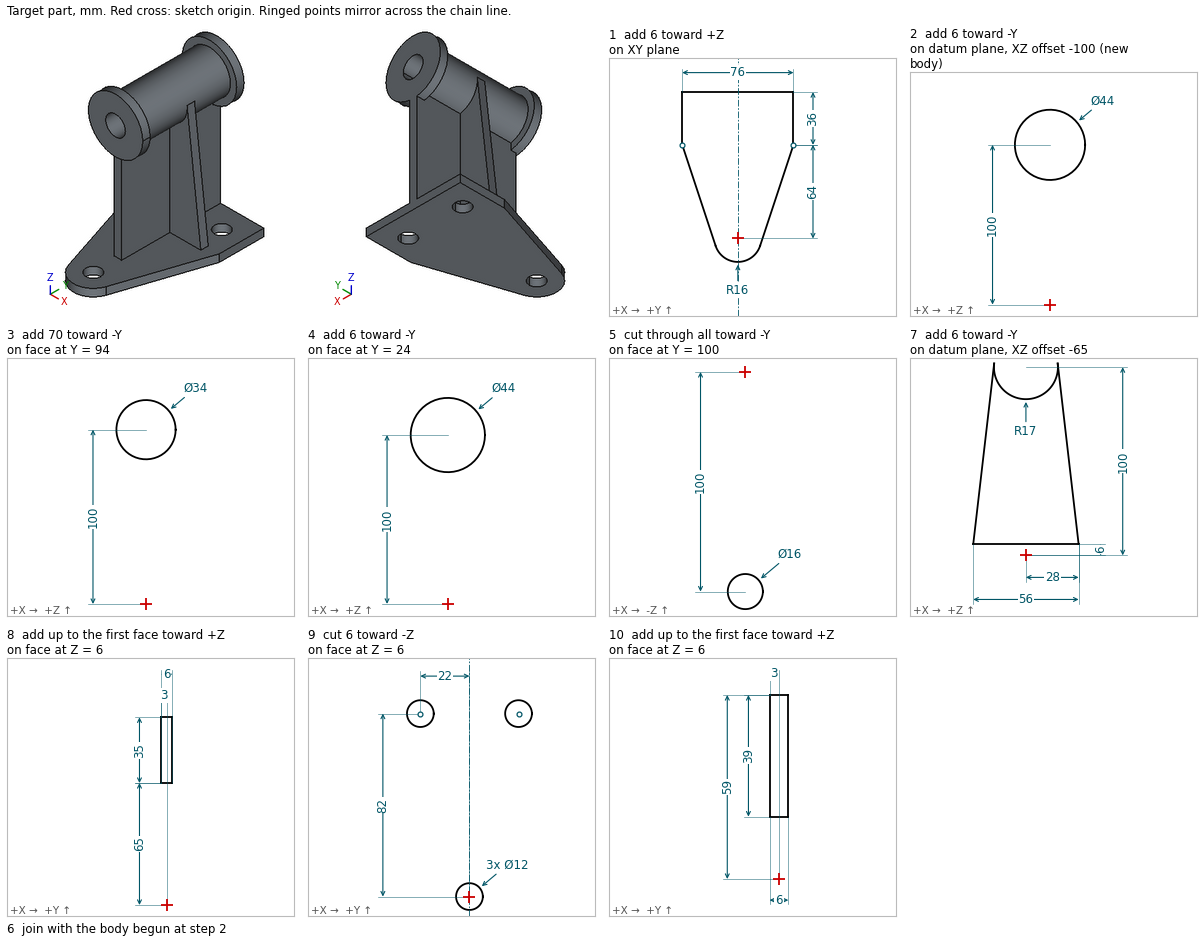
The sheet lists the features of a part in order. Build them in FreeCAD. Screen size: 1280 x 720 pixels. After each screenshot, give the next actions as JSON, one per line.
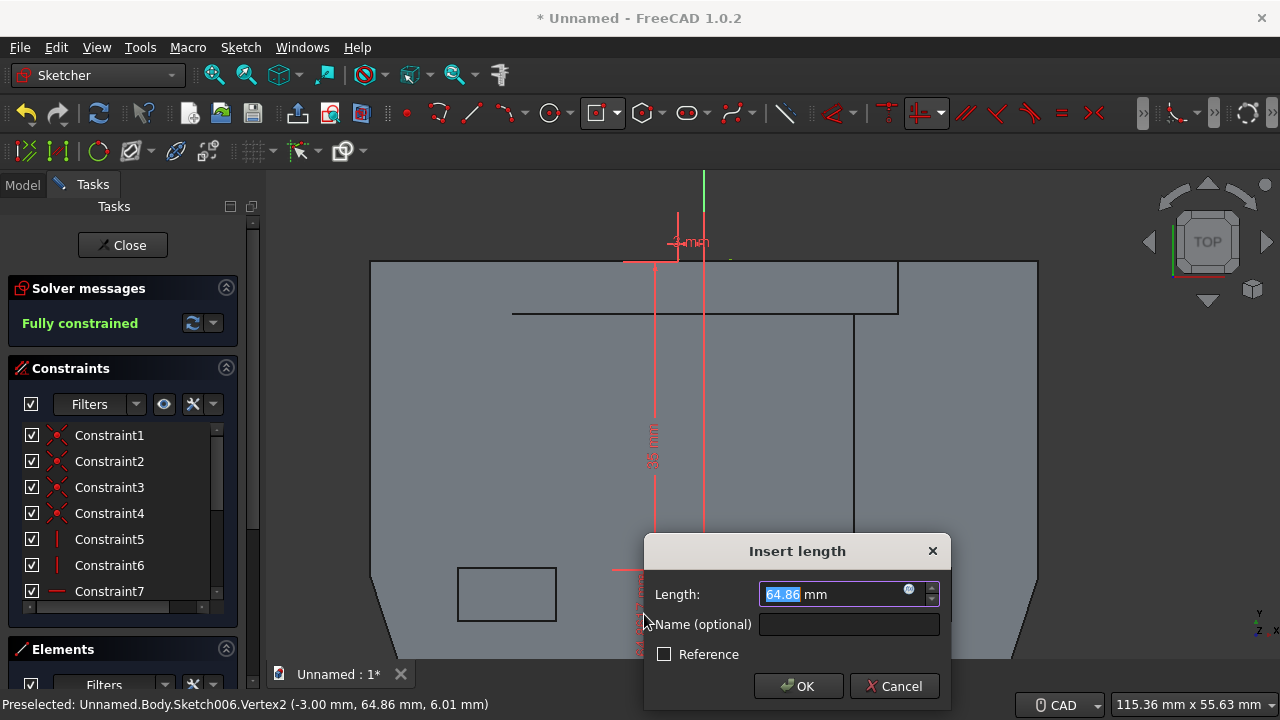
{"action": "type", "text": "65"}
{"action": "key", "text": "Return"}
{"action": "key", "text": "Escape"}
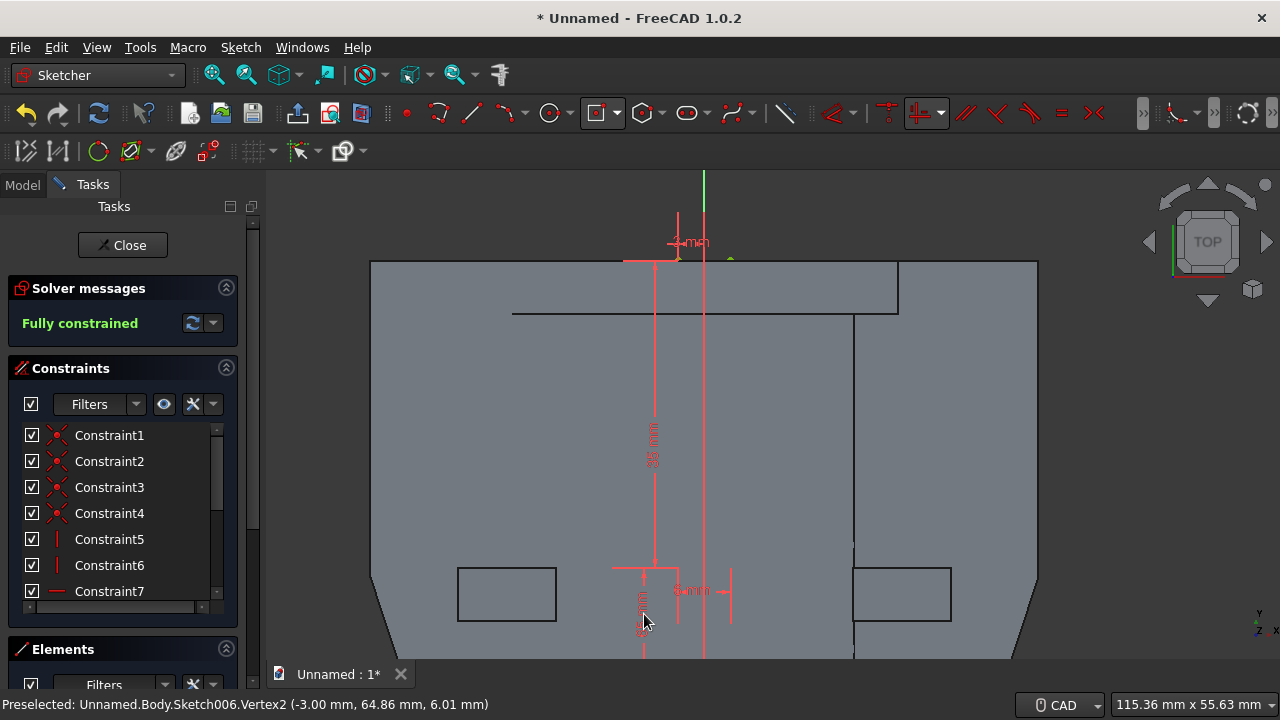
{"action": "left_click", "coordinate": [123, 245]}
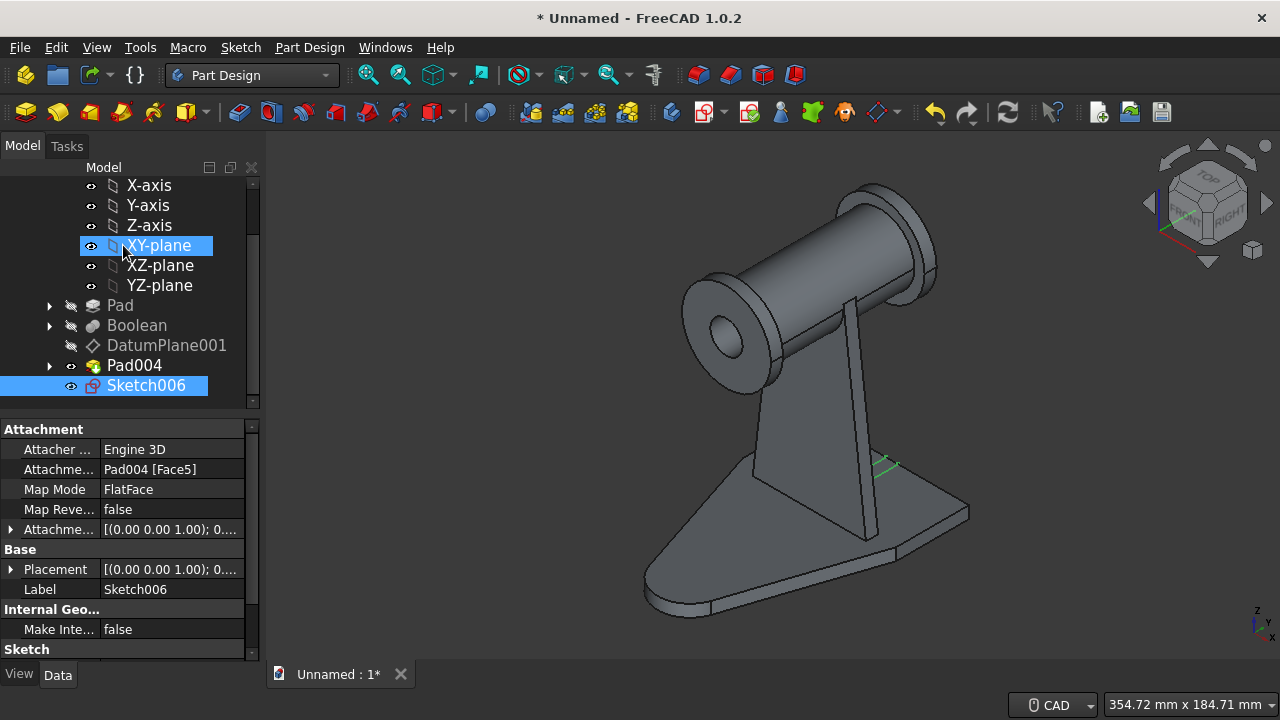
{"action": "left_click", "coordinate": [26, 112]}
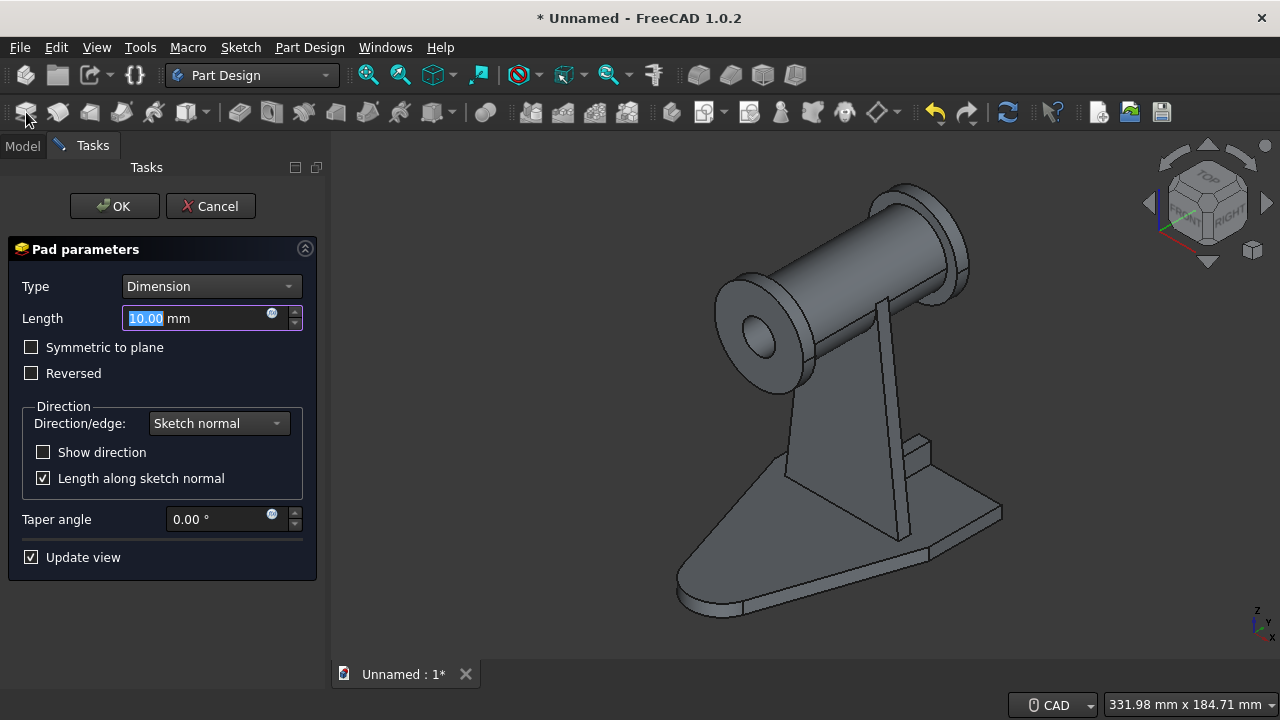
{"action": "left_click", "coordinate": [212, 286]}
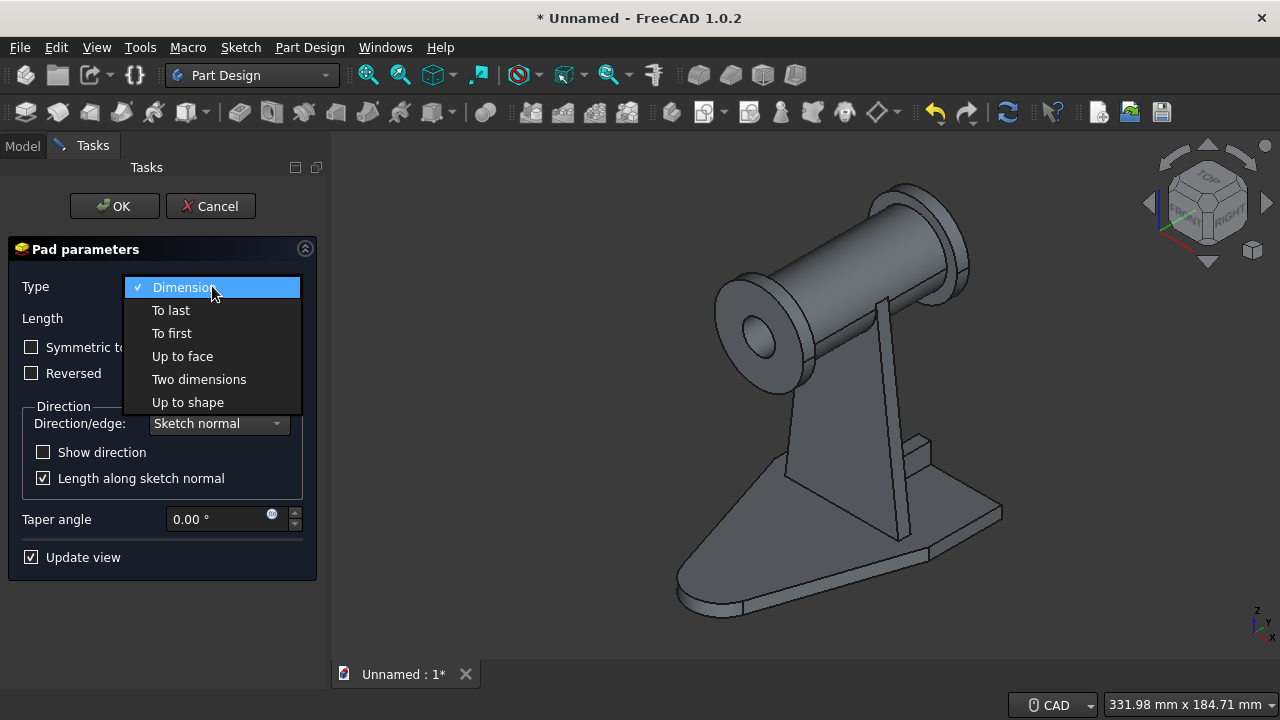
{"action": "left_click", "coordinate": [212, 334]}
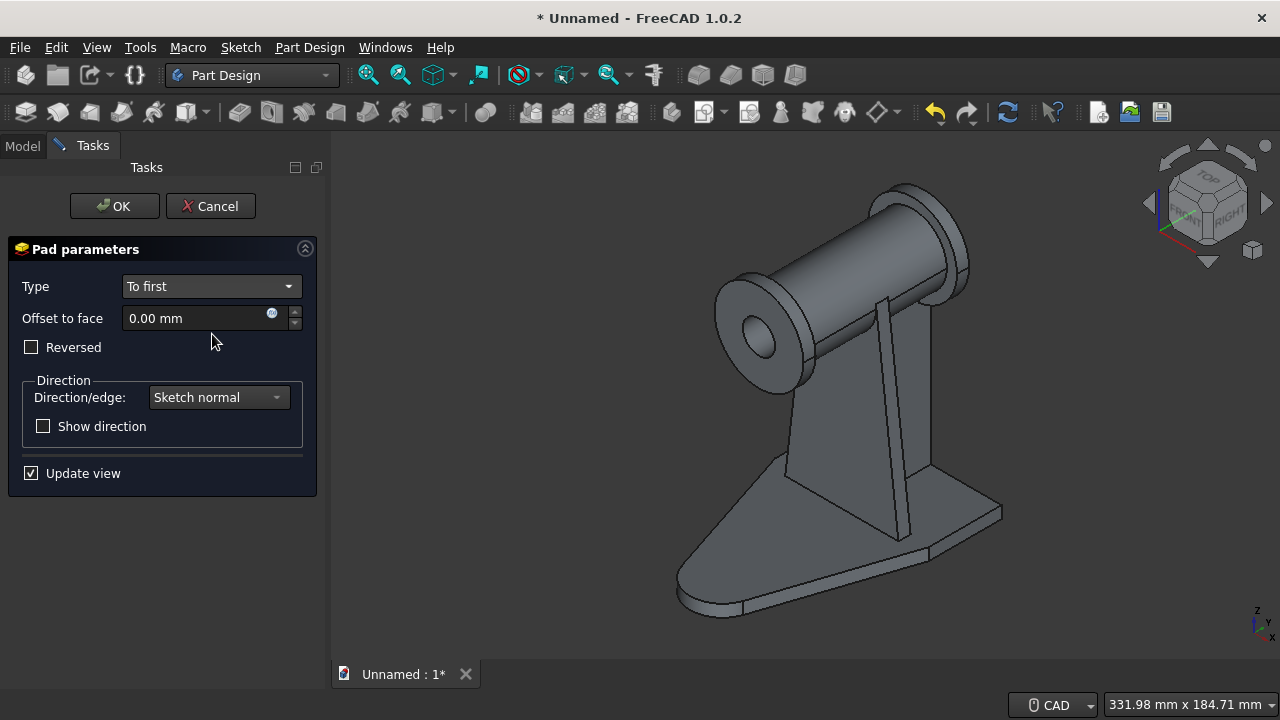
{"action": "left_click", "coordinate": [115, 206]}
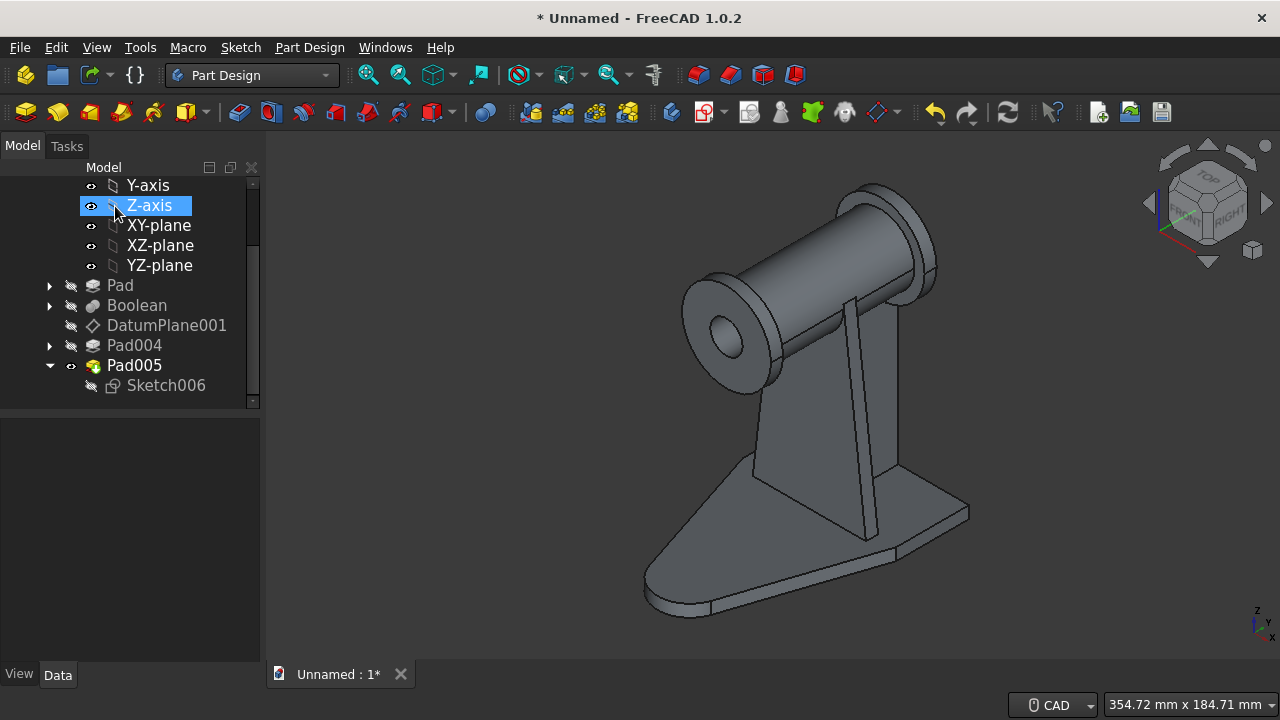
{"action": "left_click", "coordinate": [708, 566]}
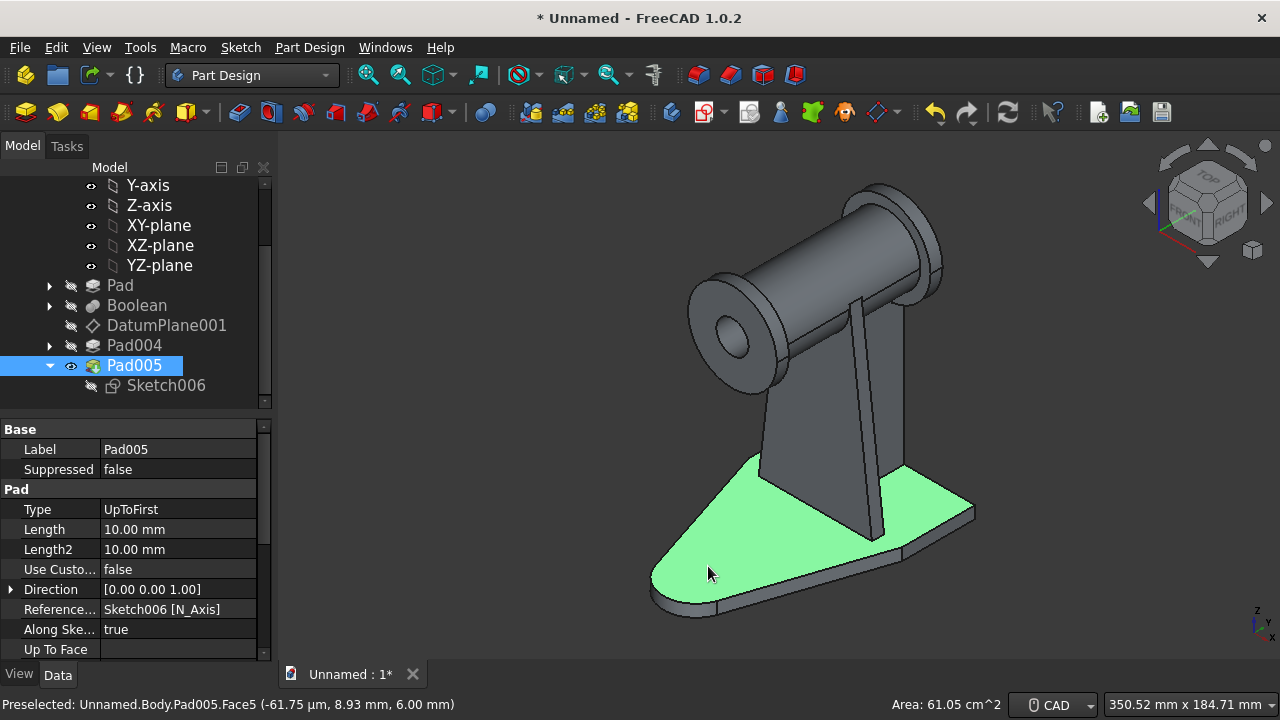
{"action": "left_click", "coordinate": [704, 112]}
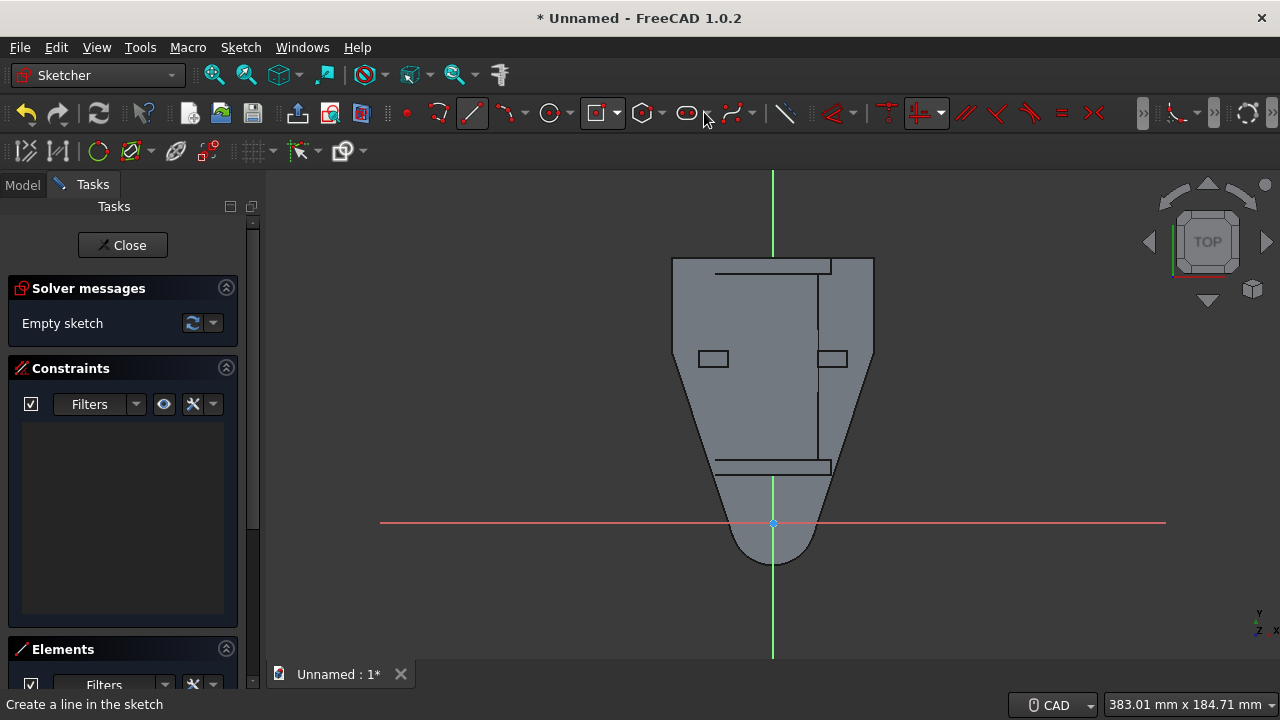
{"action": "key", "text": "q s"}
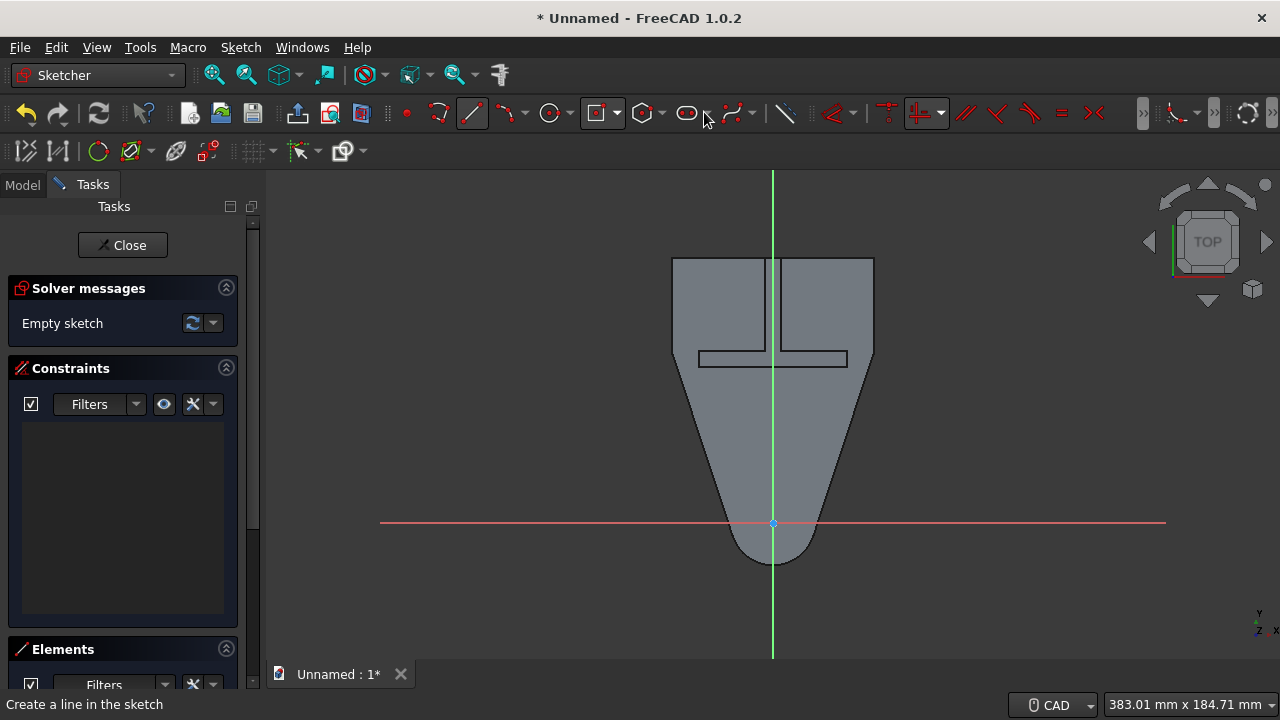
{"action": "left_click", "coordinate": [550, 114]}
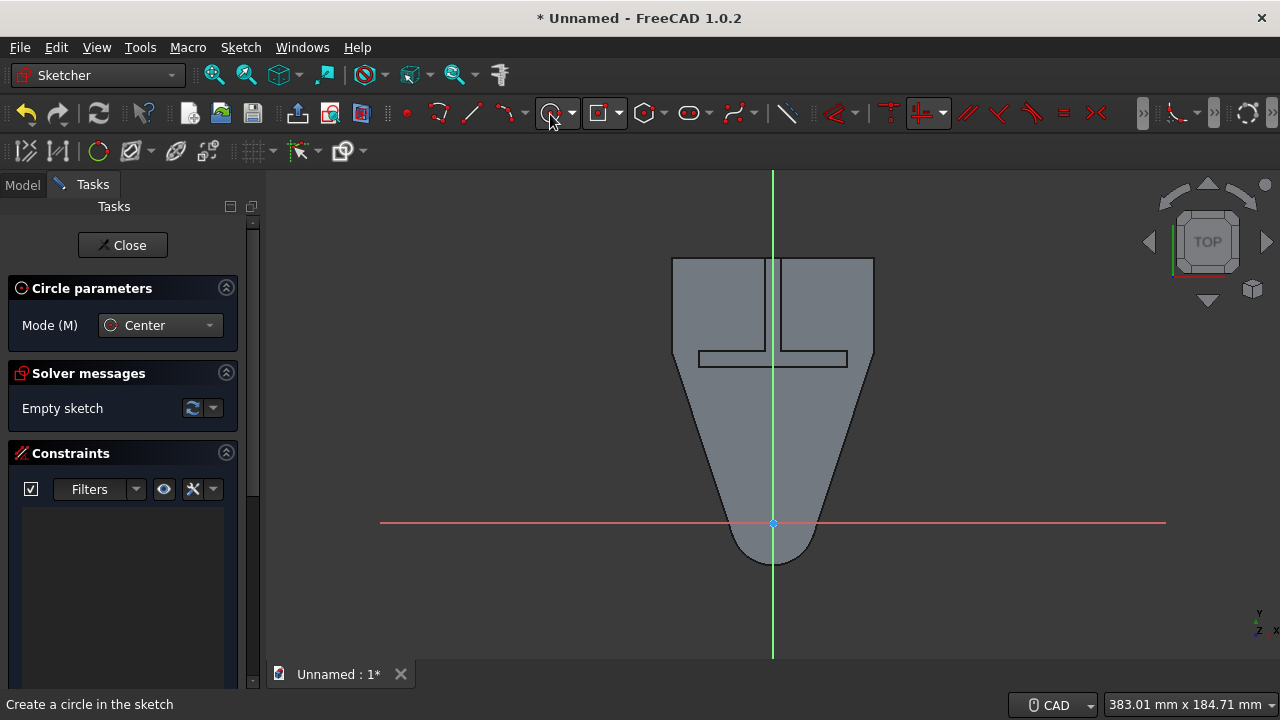
{"action": "scroll", "coordinate": [773, 523], "scroll_direction": "up", "scroll_amount": 2}